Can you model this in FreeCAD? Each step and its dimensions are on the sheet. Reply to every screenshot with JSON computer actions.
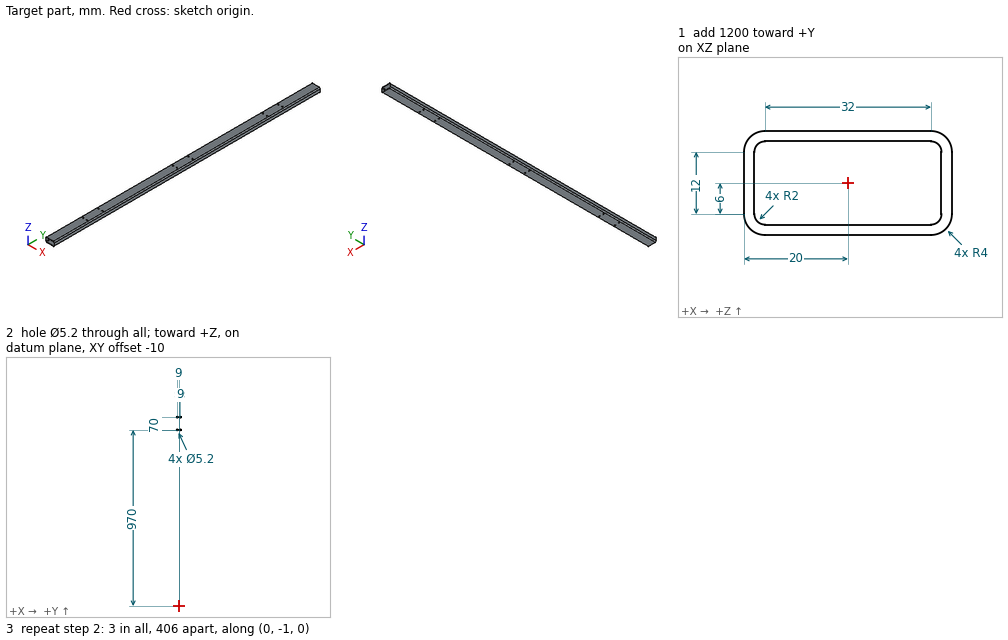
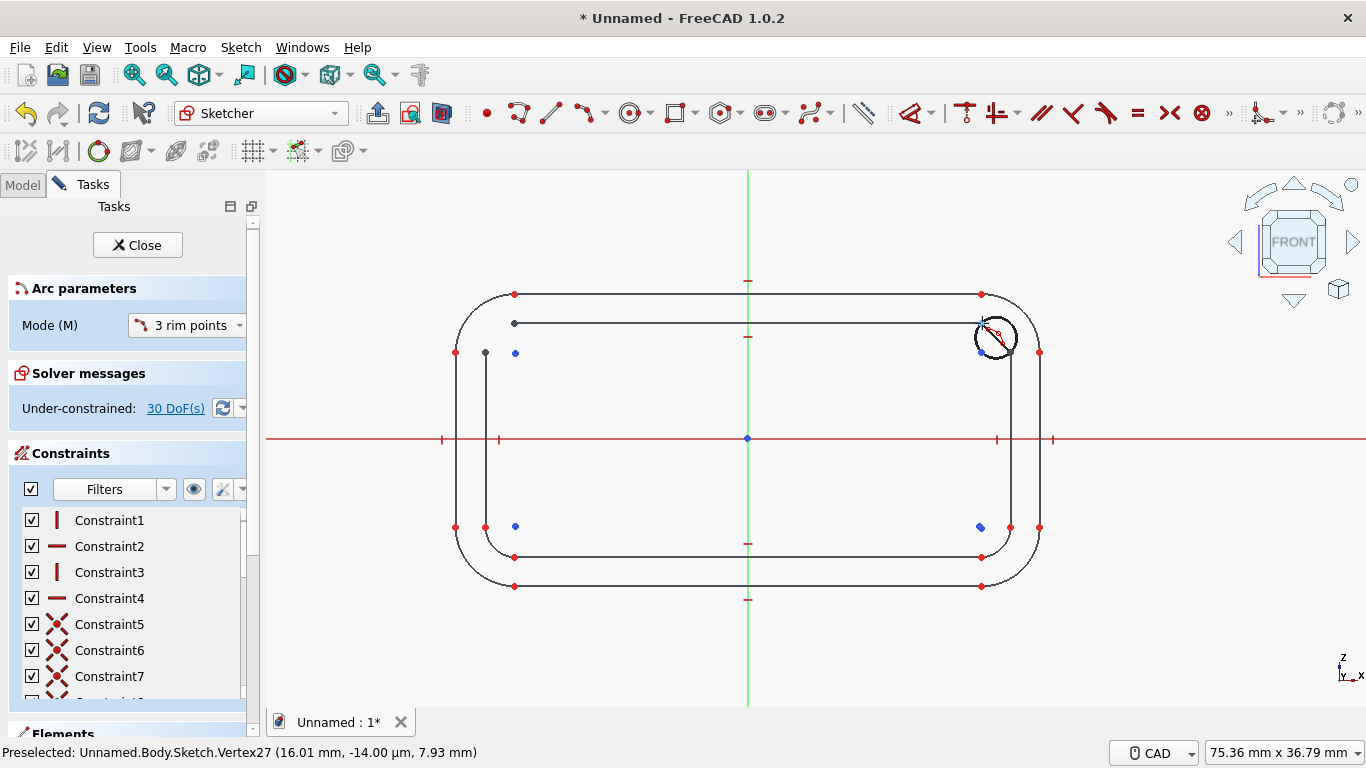
{"action": "scroll", "coordinate": [1002, 331], "scroll_direction": "up", "scroll_amount": 4}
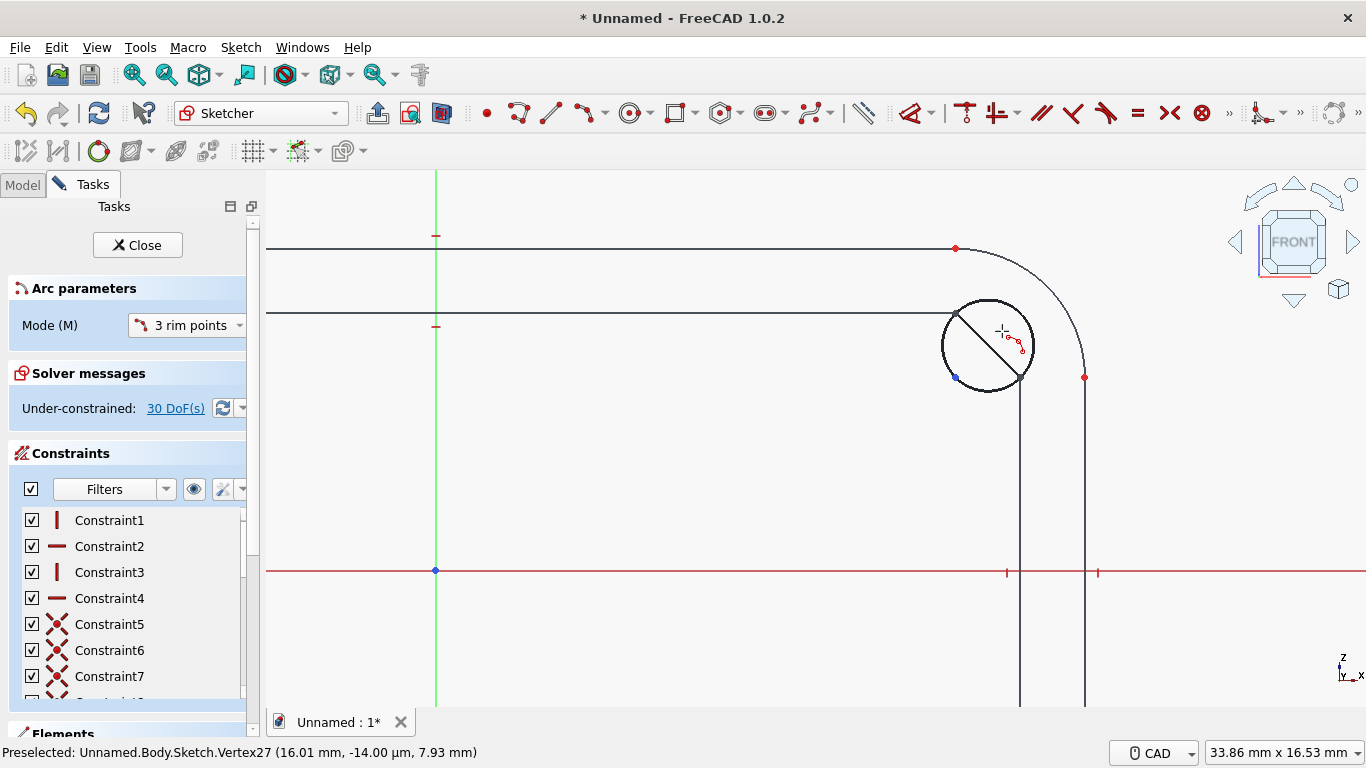
{"action": "left_click", "coordinate": [1002, 330]}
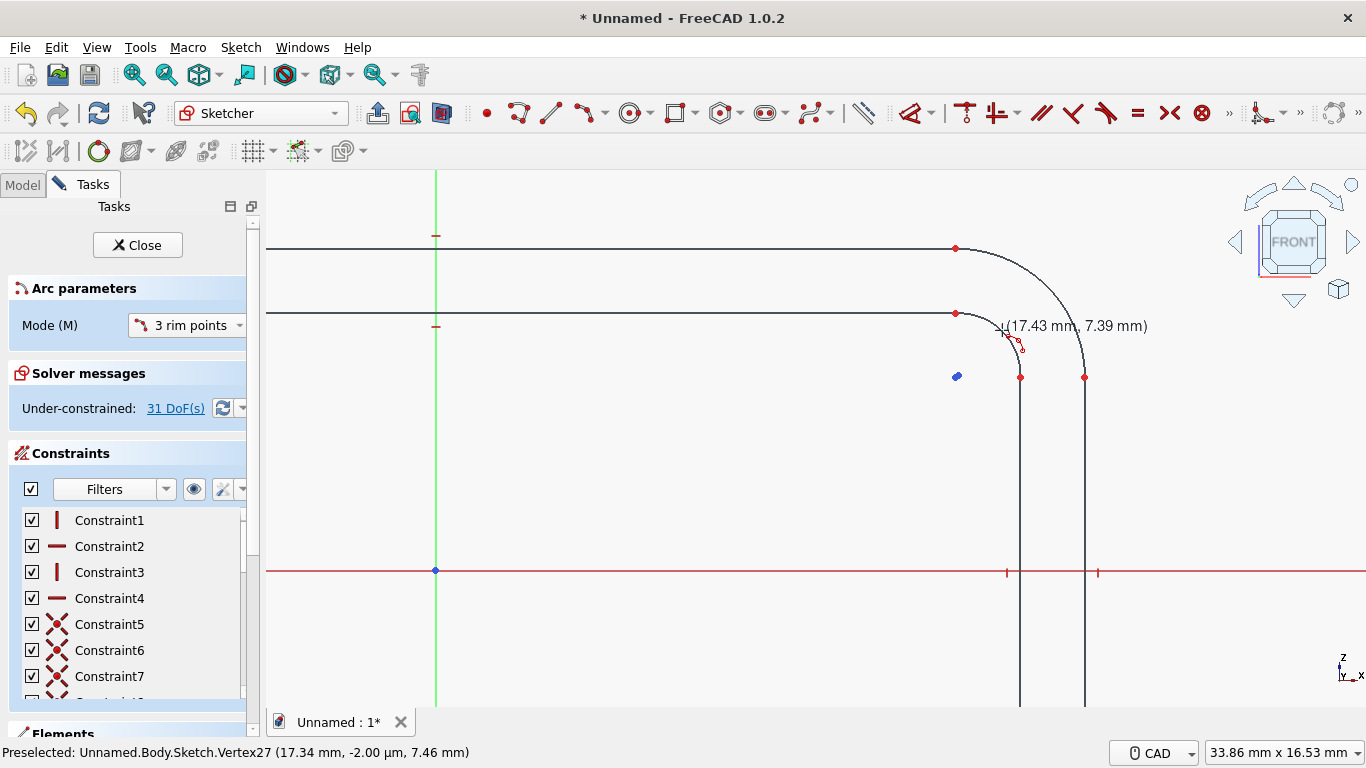
{"action": "scroll", "coordinate": [1002, 330], "scroll_direction": "down", "scroll_amount": 4}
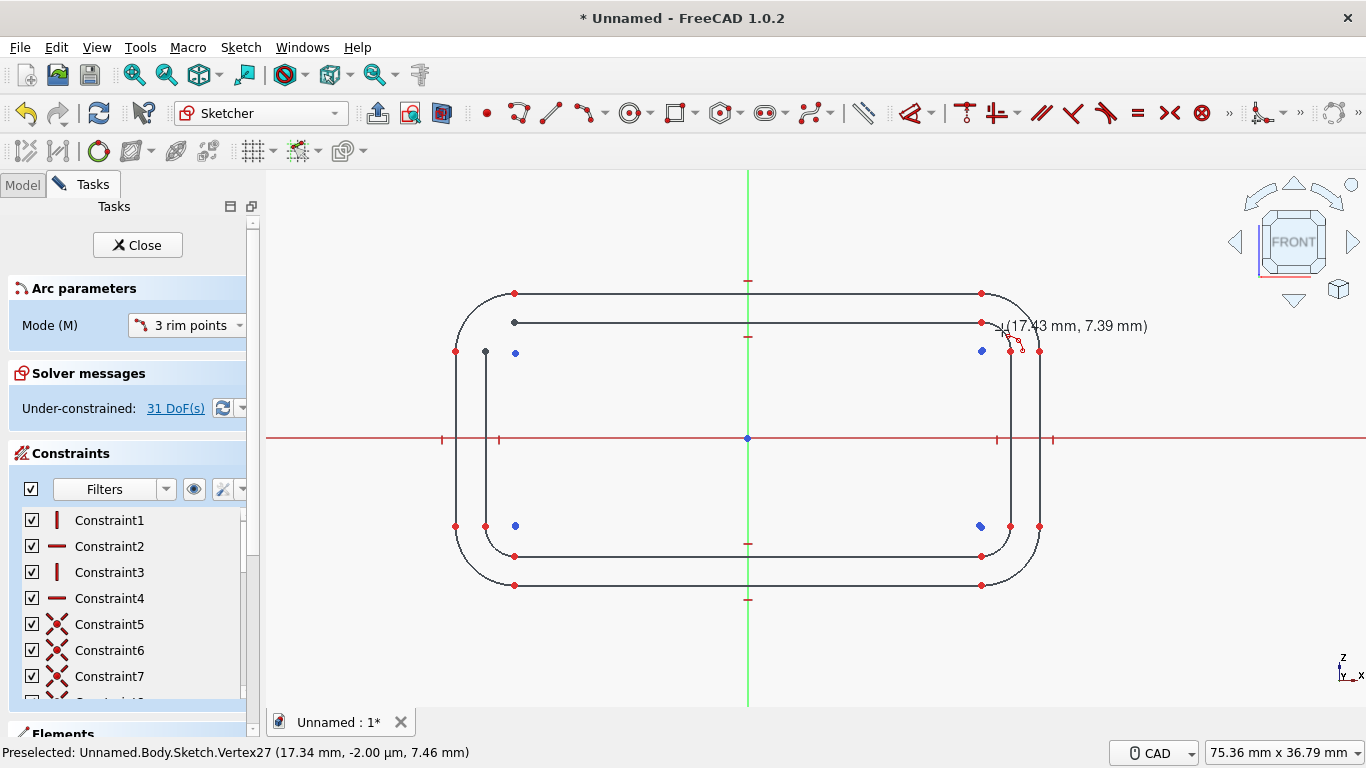
{"action": "left_click", "coordinate": [515, 323]}
{"action": "left_click", "coordinate": [486, 352]}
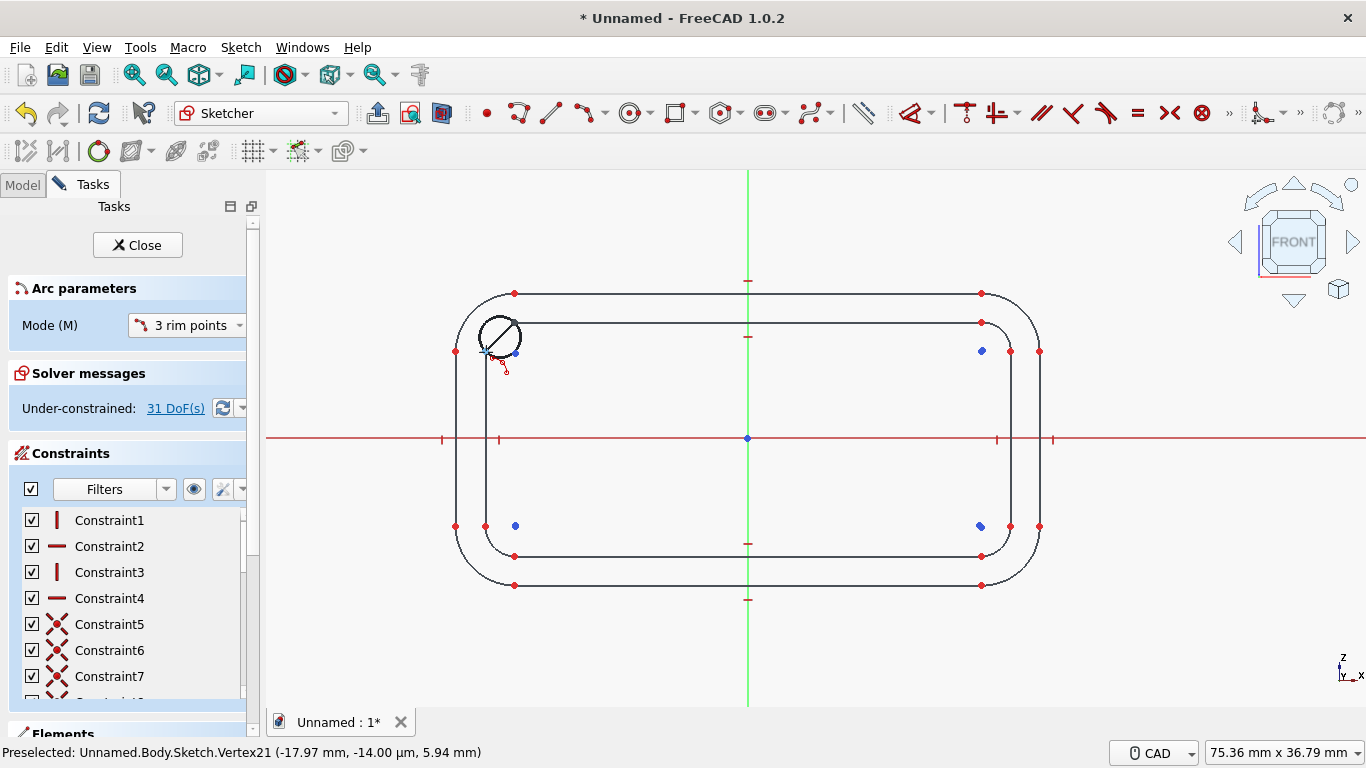
{"action": "scroll", "coordinate": [494, 330], "scroll_direction": "up", "scroll_amount": 4}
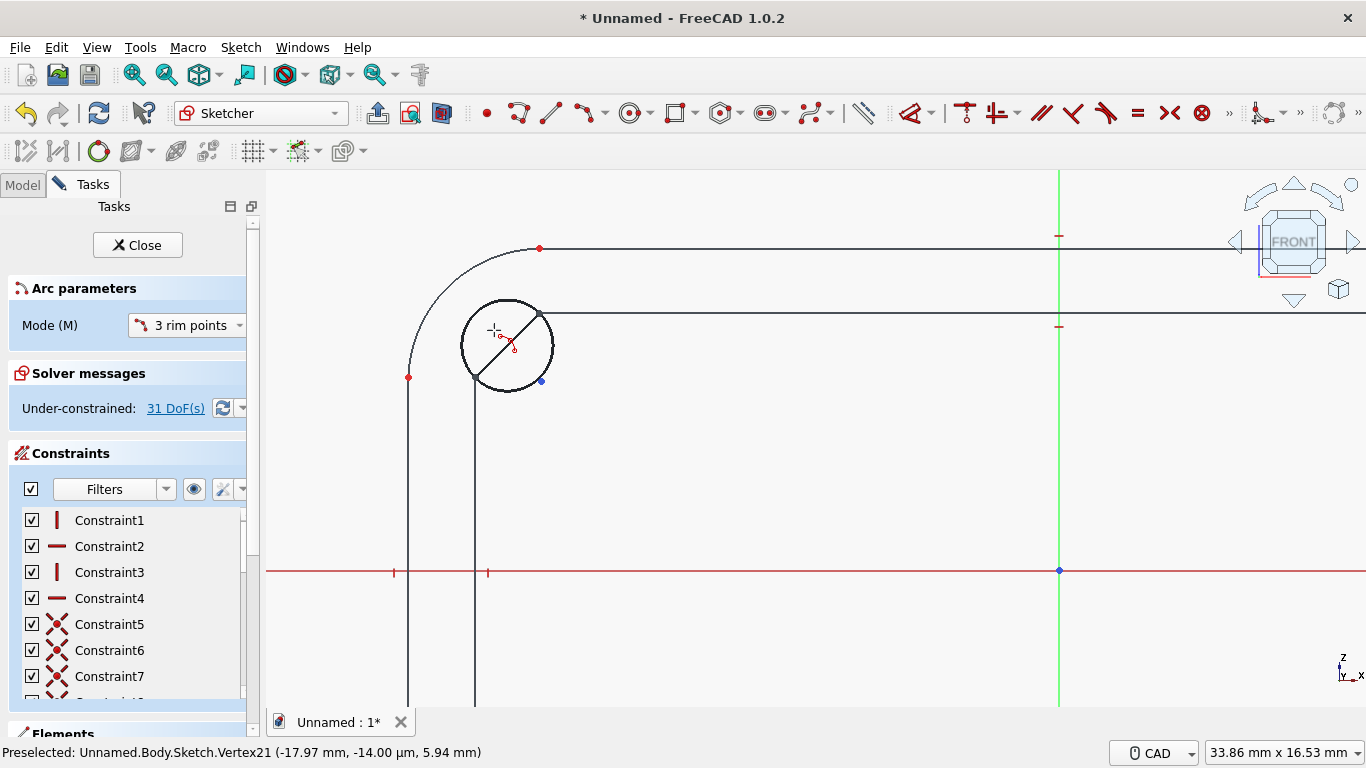
{"action": "left_click", "coordinate": [493, 330]}
{"action": "key", "text": "Escape"}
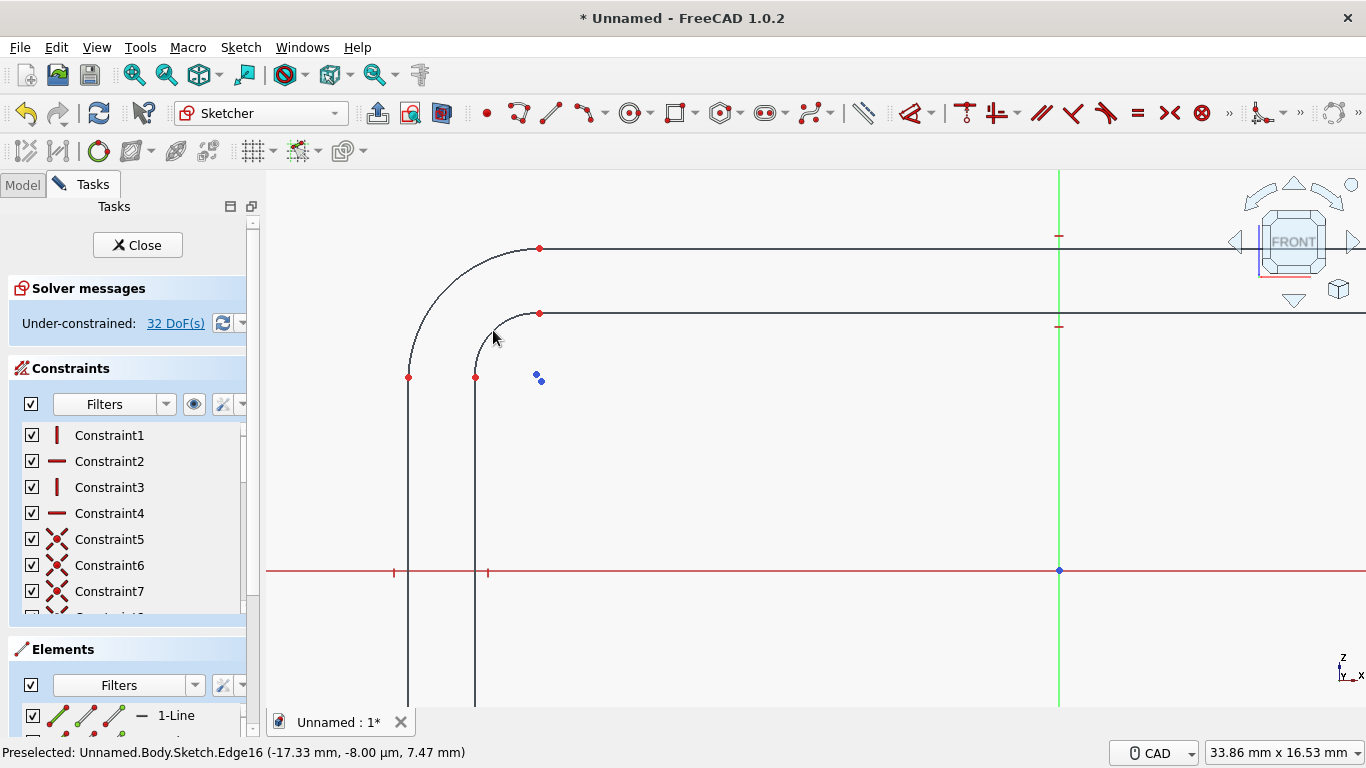
{"action": "left_click", "coordinate": [408, 650]}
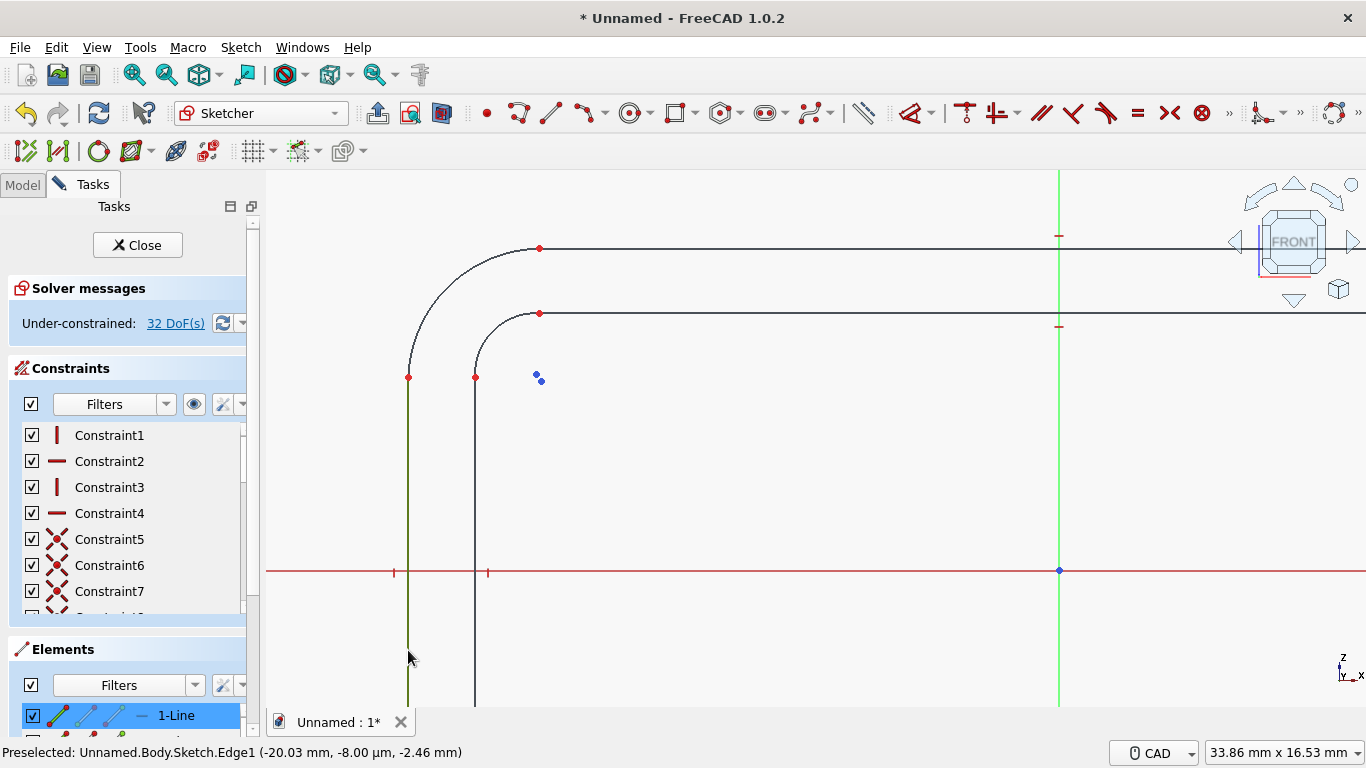
{"action": "left_click", "coordinate": [481, 263]}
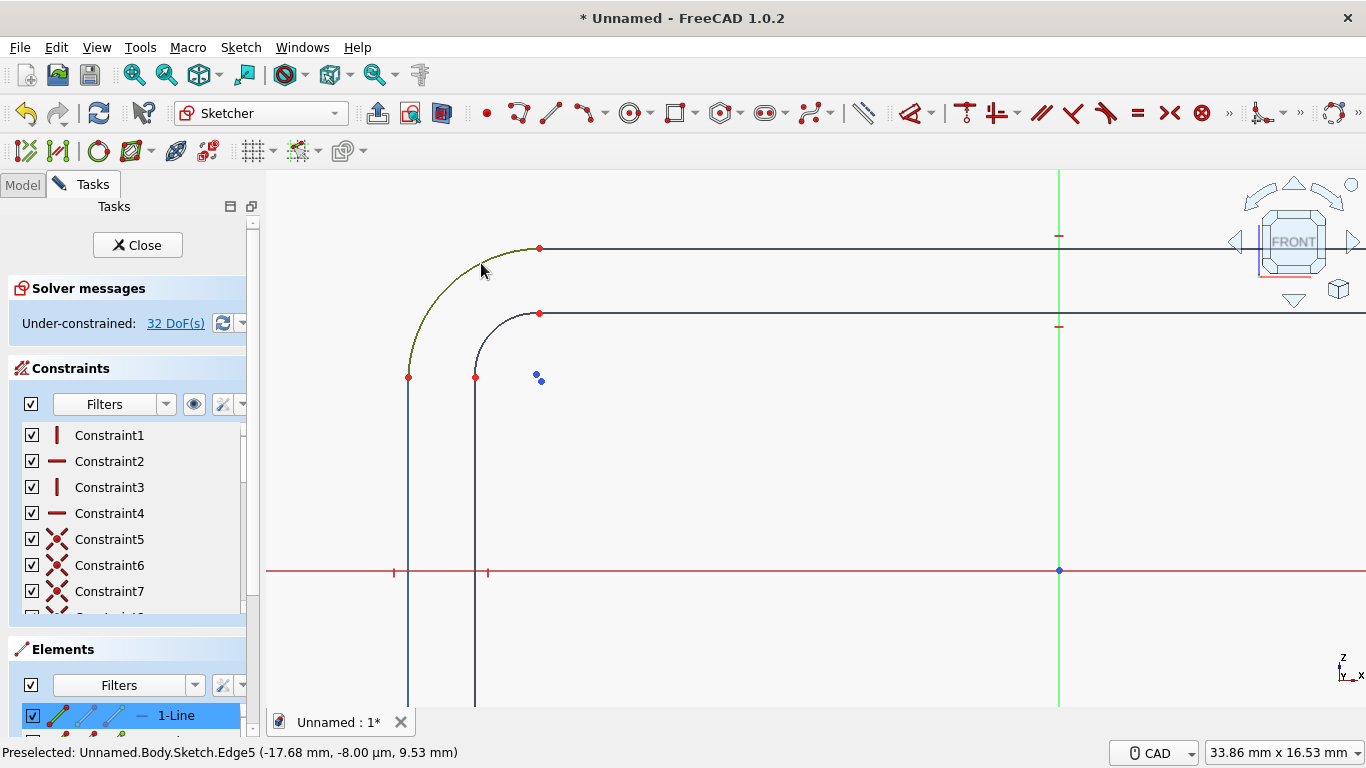
{"action": "left_click", "coordinate": [1106, 114]}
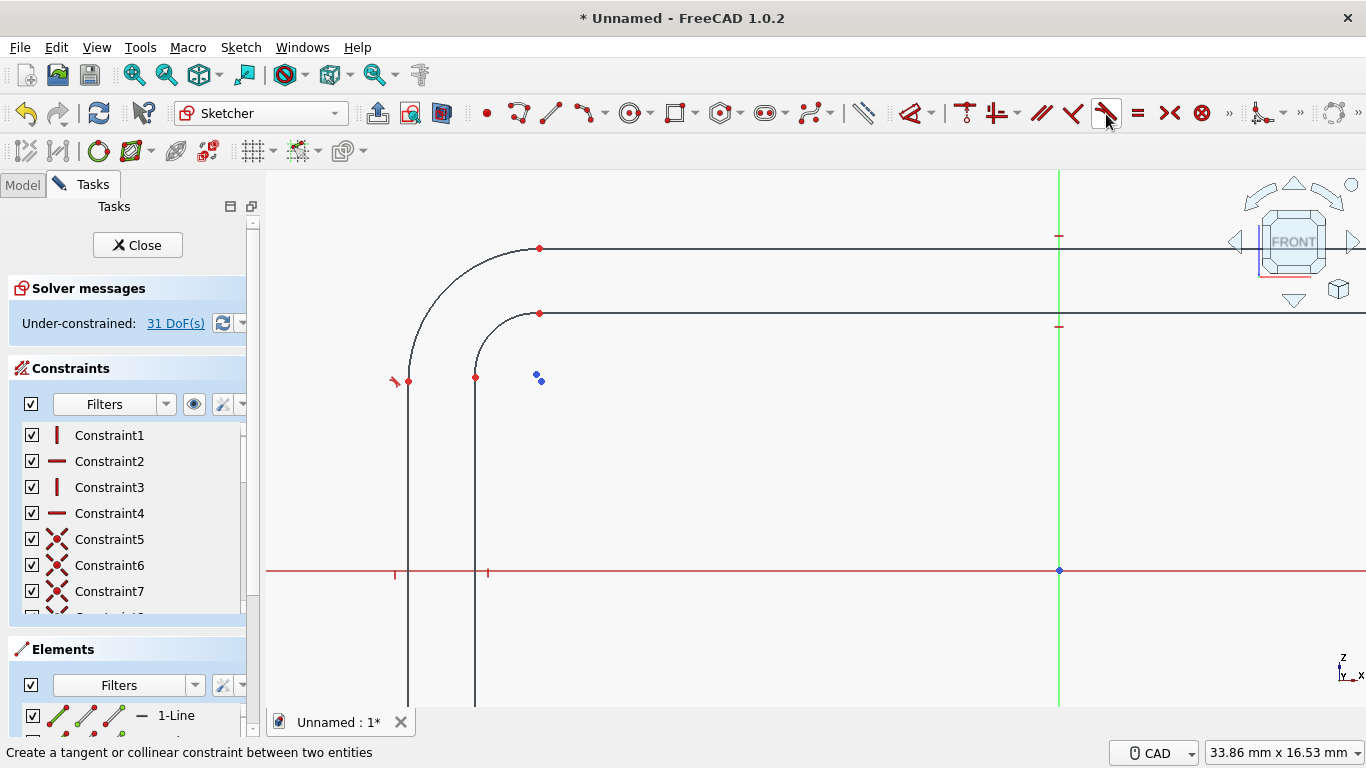
{"action": "left_click", "coordinate": [408, 652]}